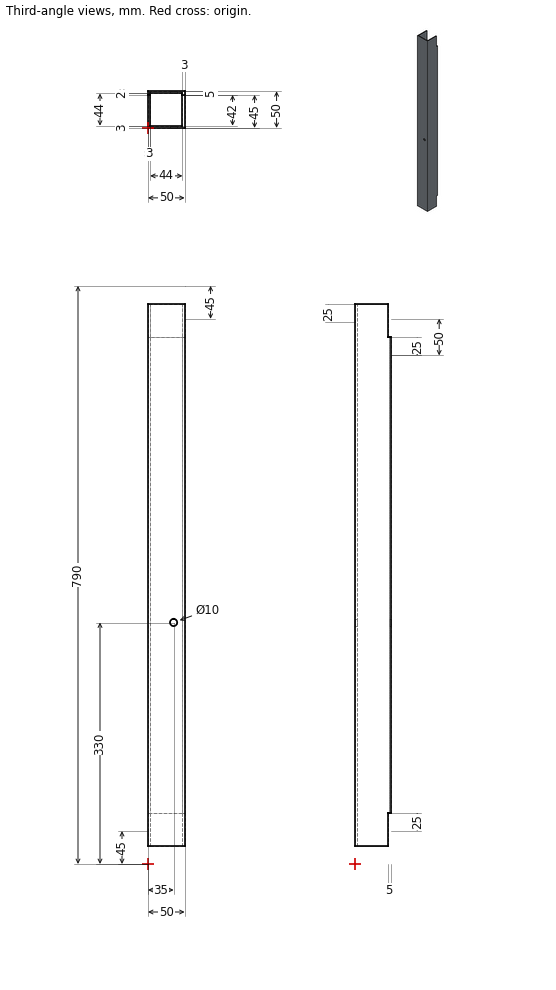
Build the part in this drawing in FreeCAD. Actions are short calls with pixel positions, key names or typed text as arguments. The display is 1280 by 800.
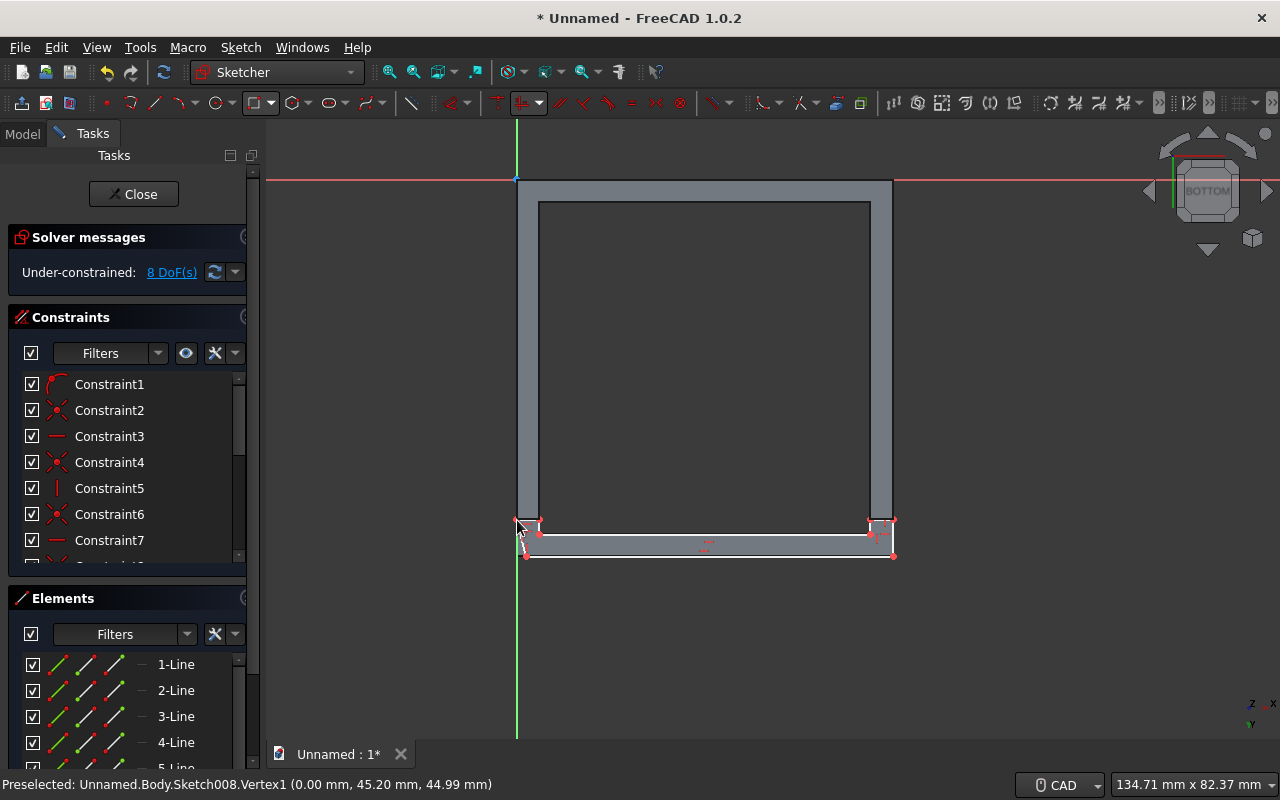
scroll(519, 531, up, 2)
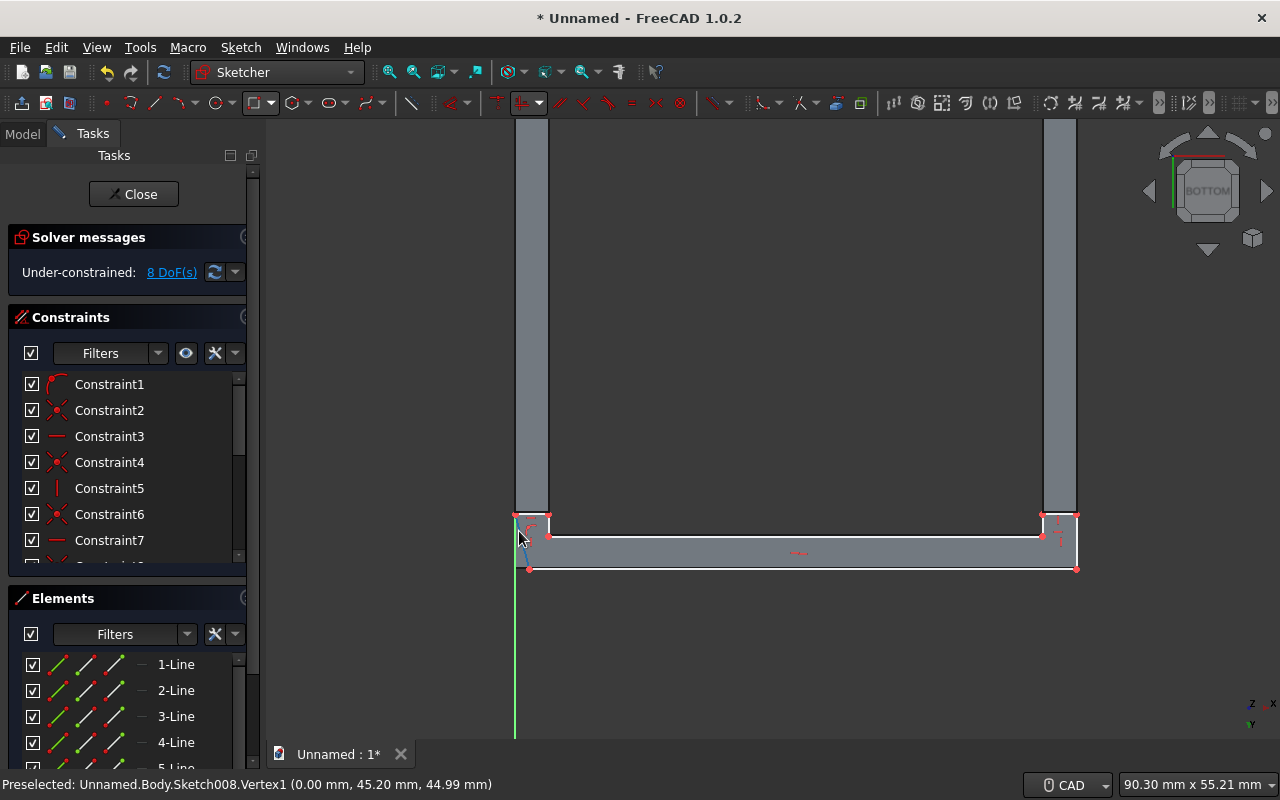
click(519, 531)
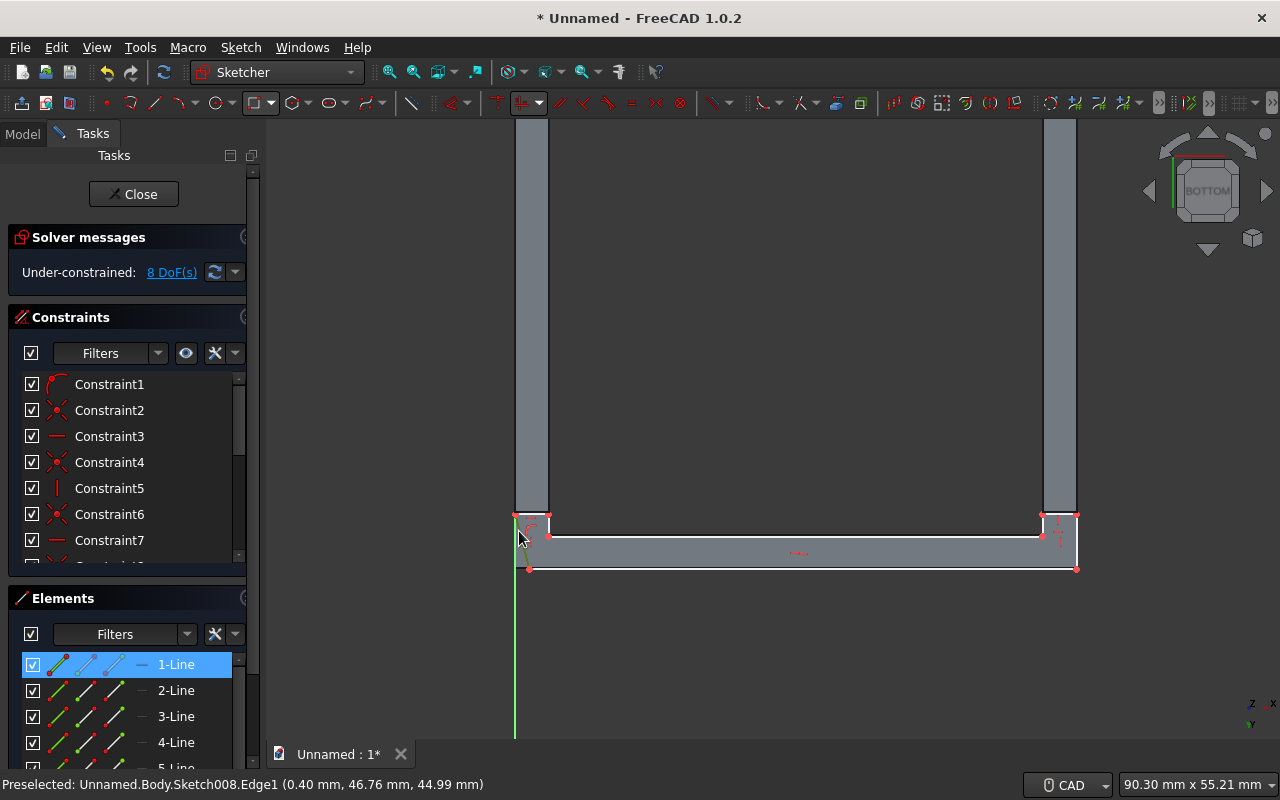
click(542, 104)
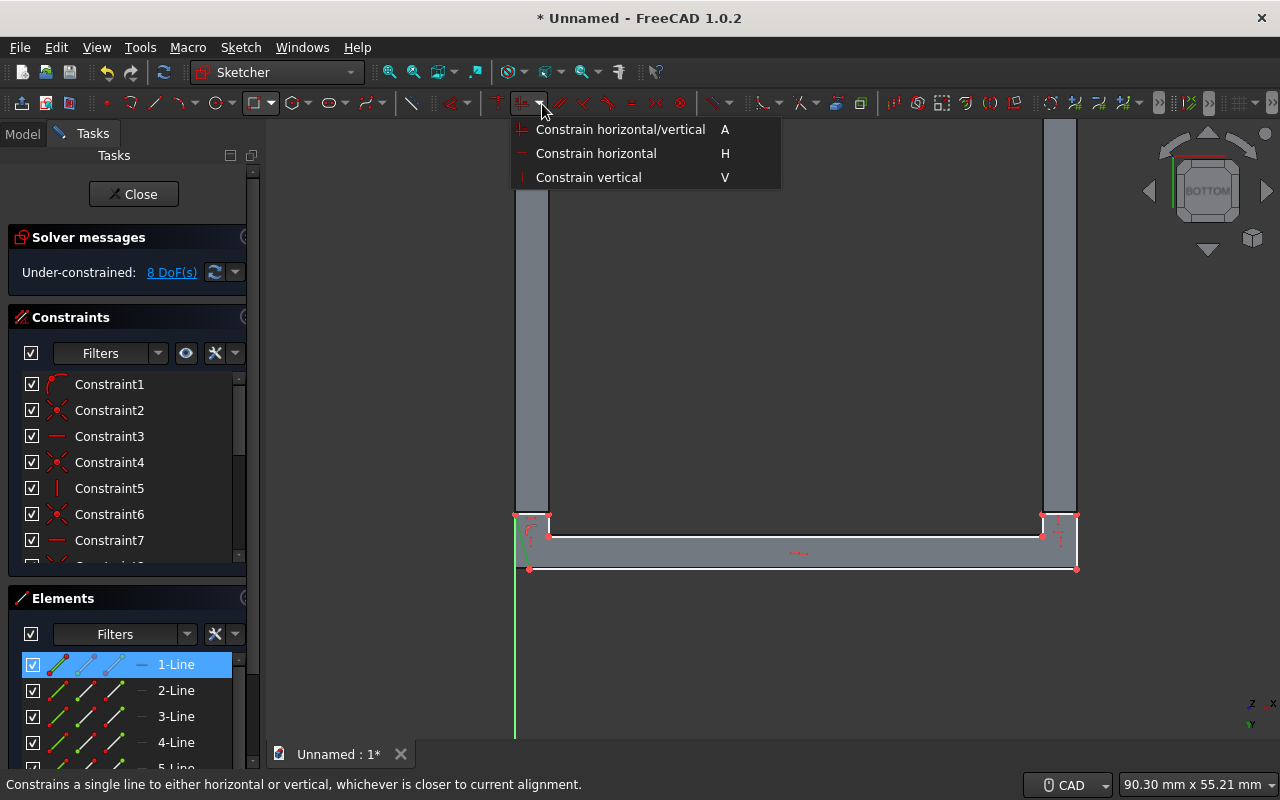
click(646, 177)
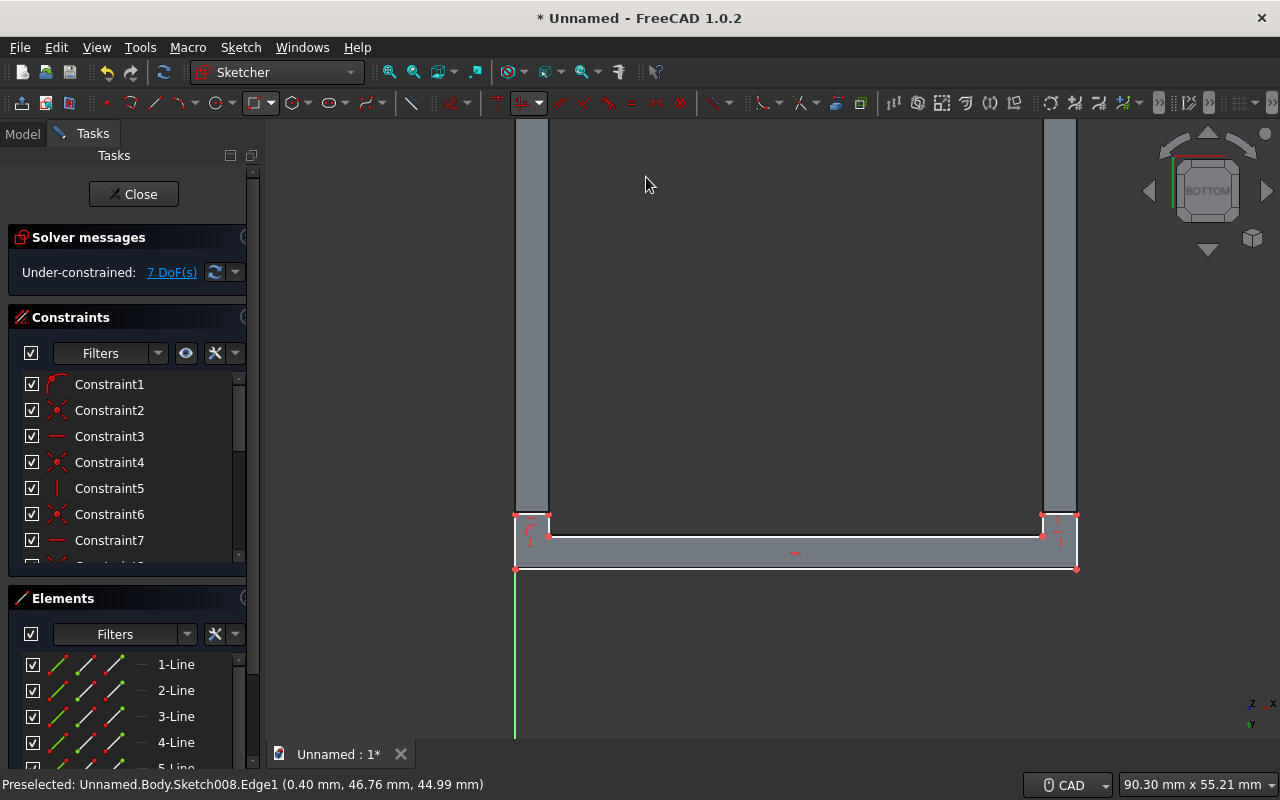
key(d)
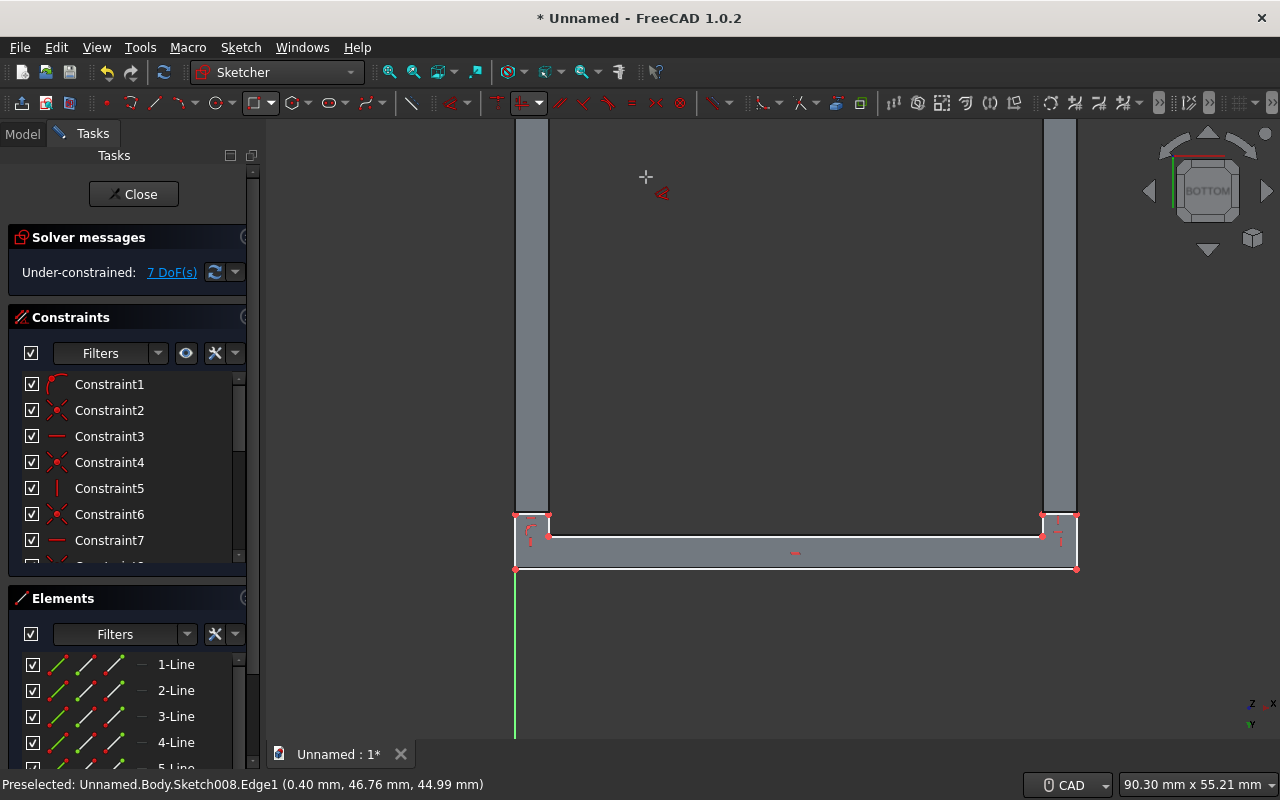
click(515, 531)
click(481, 542)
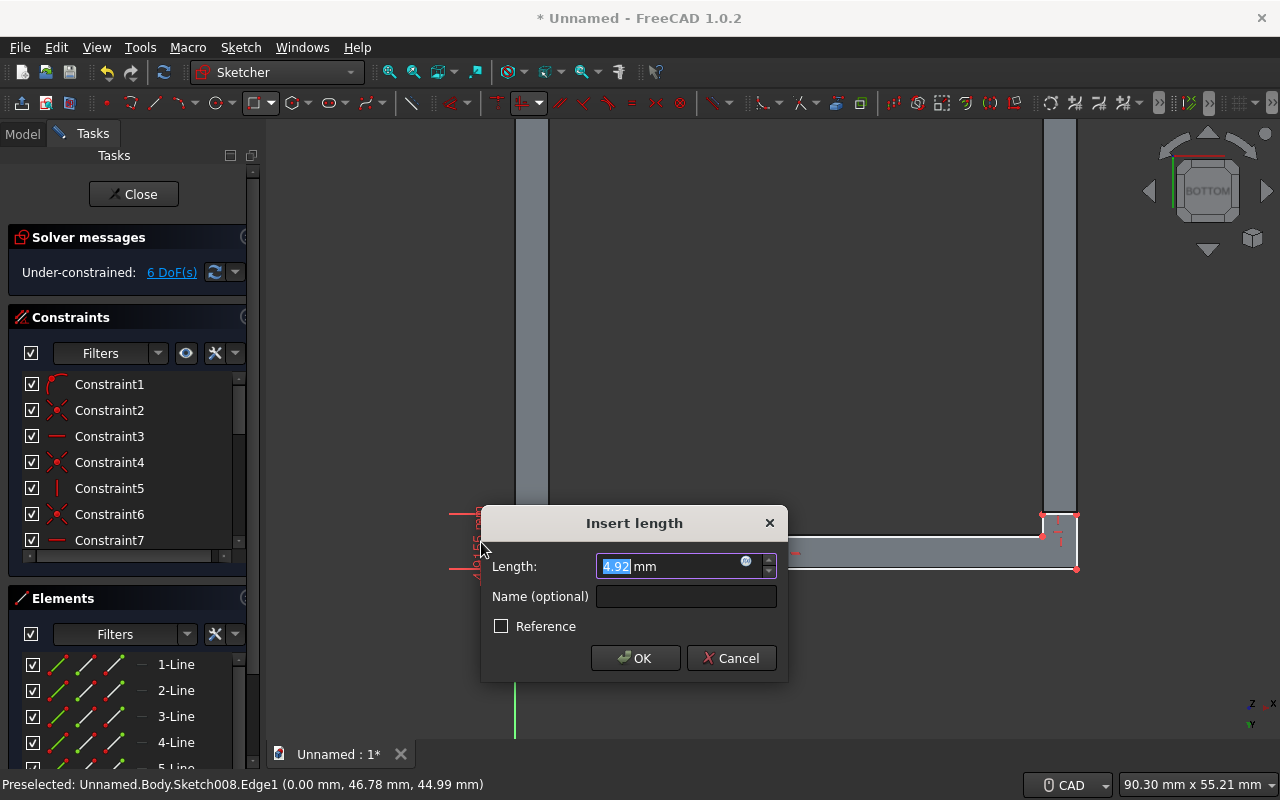
text(5)
key(Return)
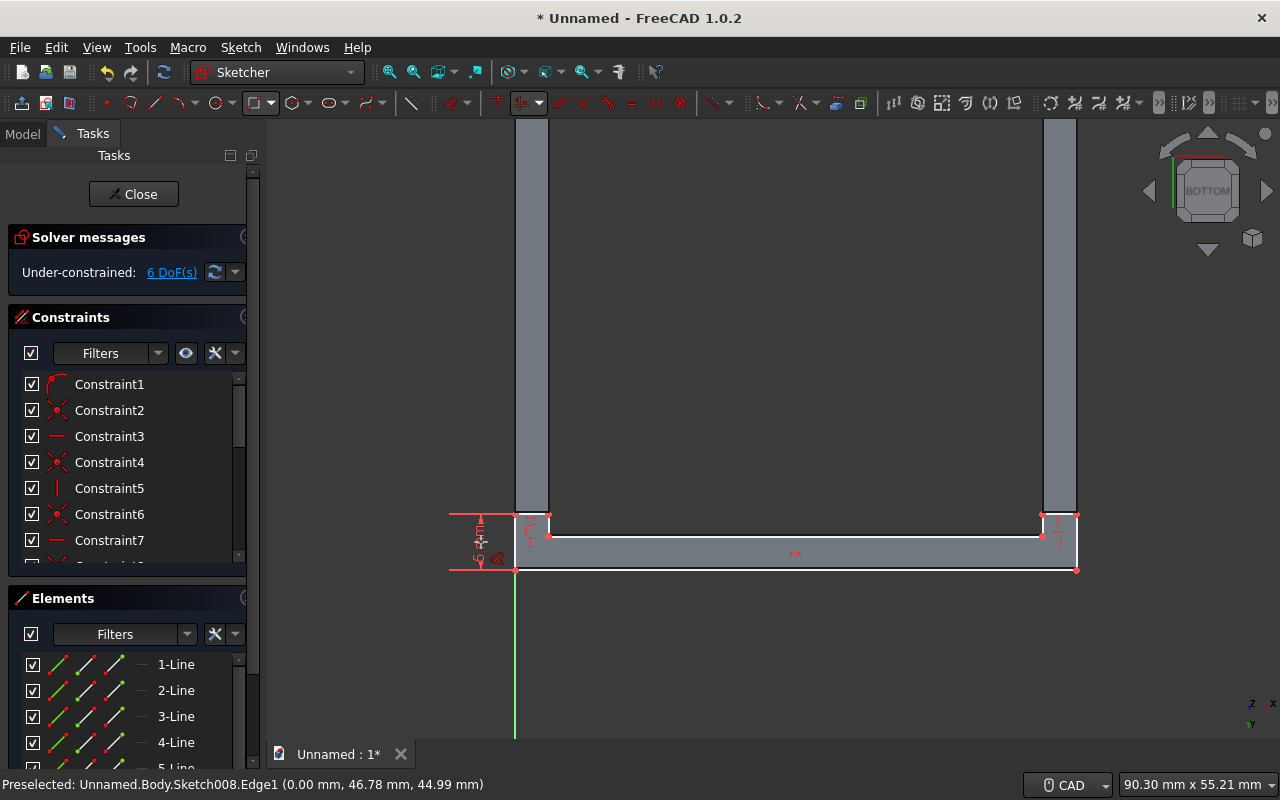
click(1077, 554)
click(1111, 542)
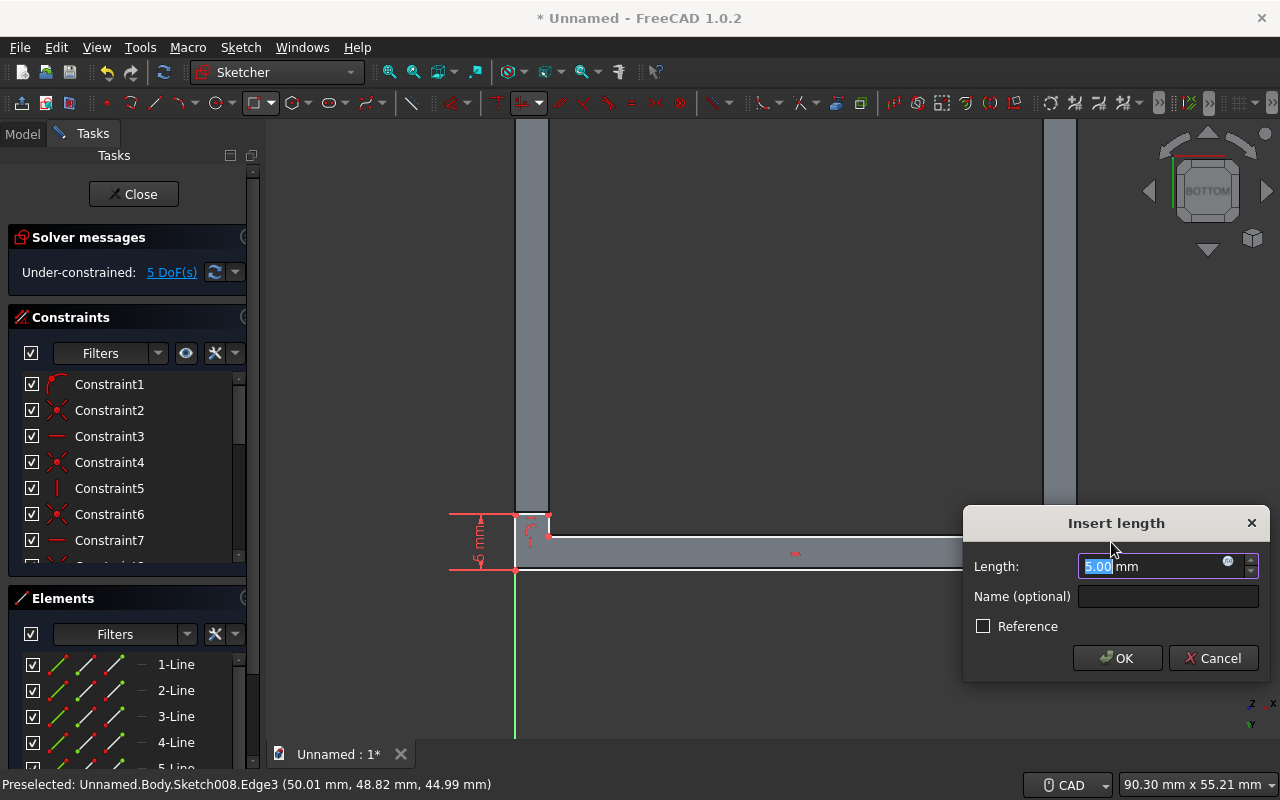
text(5)
key(Return)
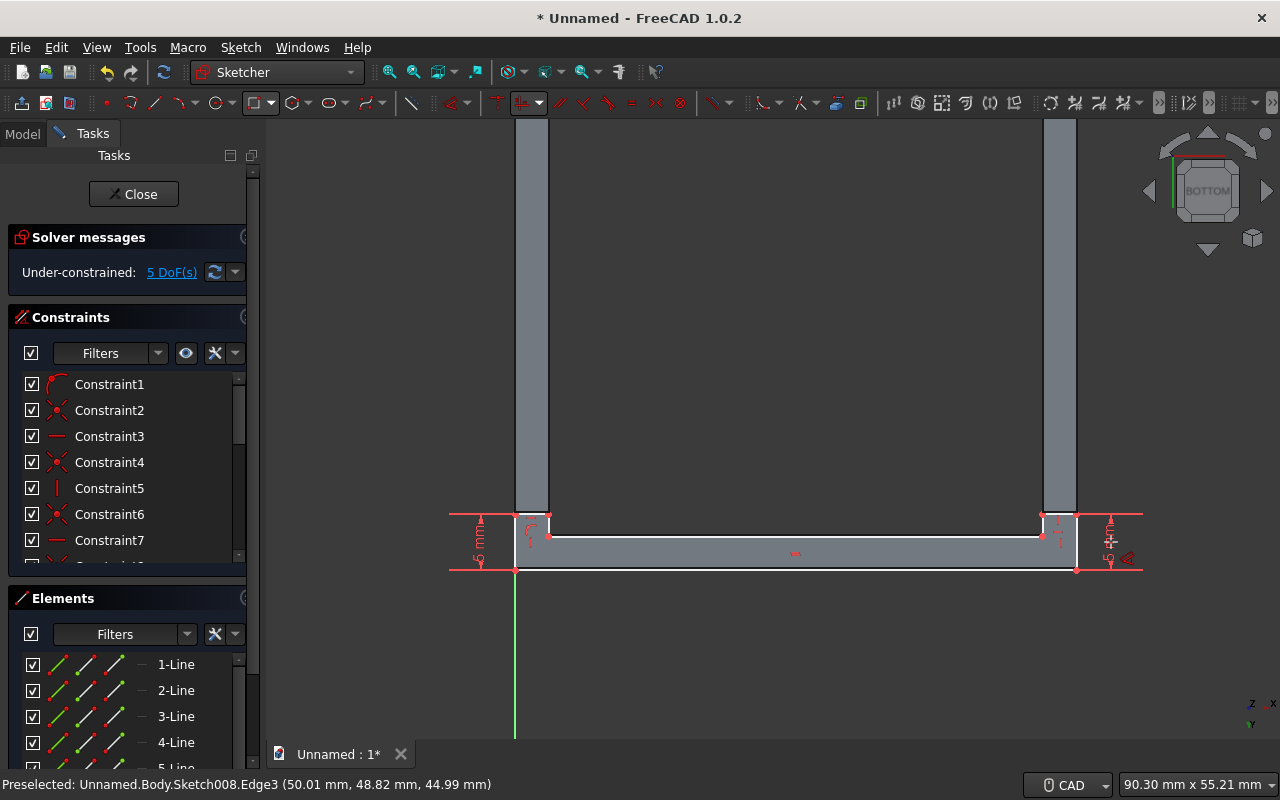
scroll(1067, 514, up, 2)